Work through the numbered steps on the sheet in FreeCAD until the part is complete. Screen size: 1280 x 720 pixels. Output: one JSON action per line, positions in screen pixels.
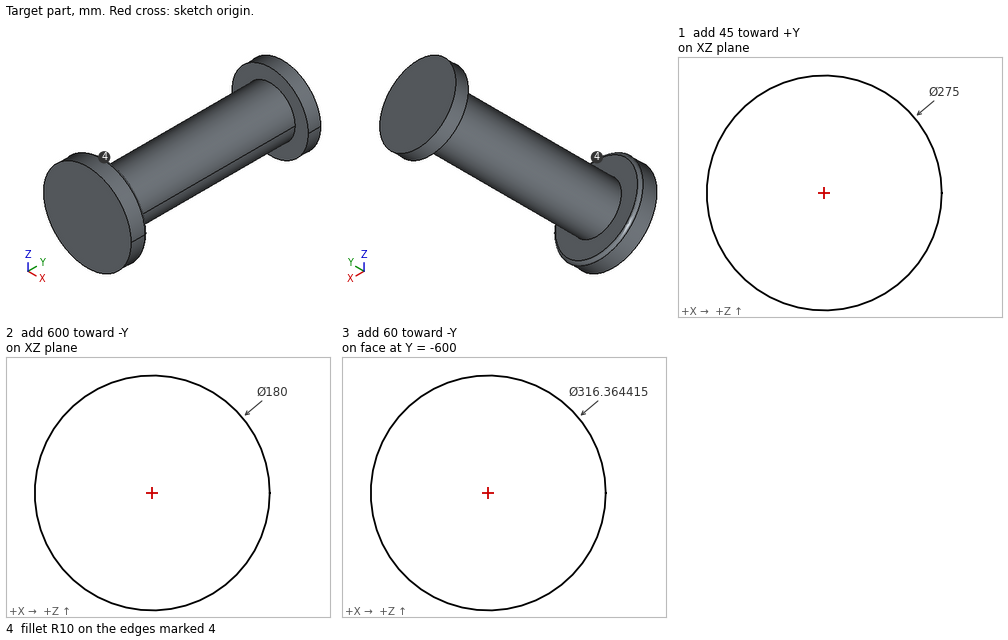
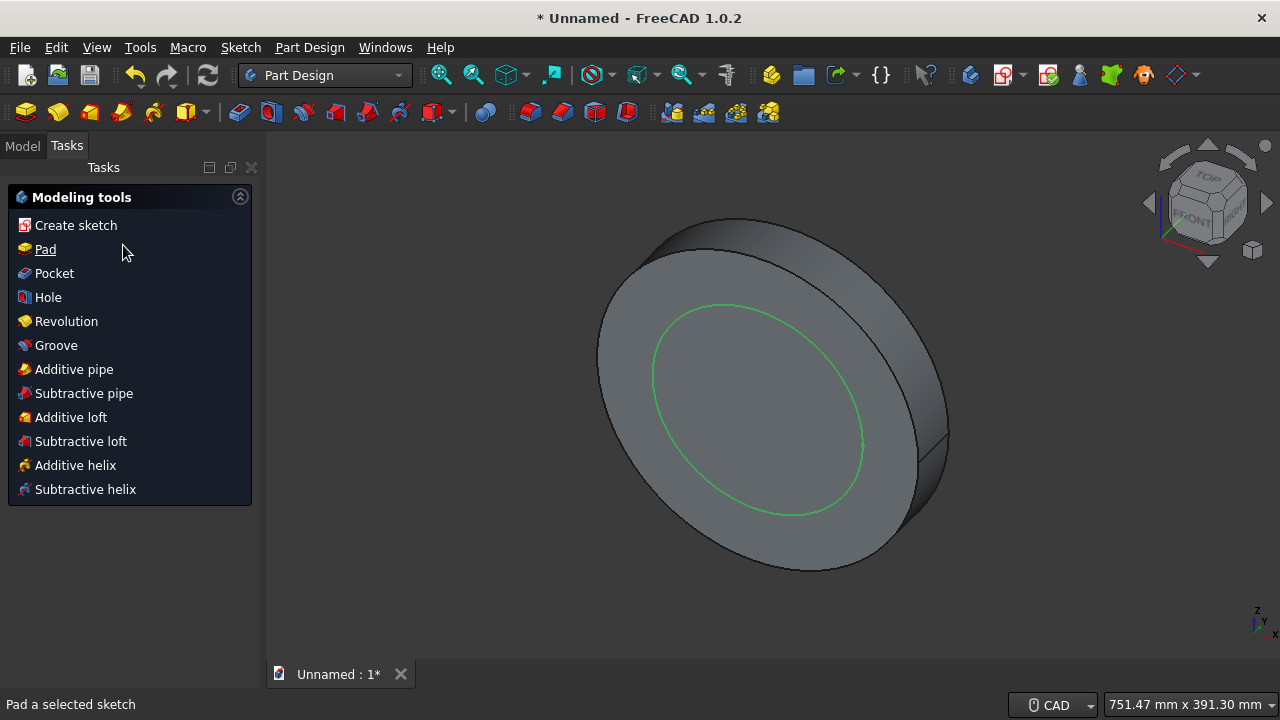
{"action": "left_click", "coordinate": [26, 112]}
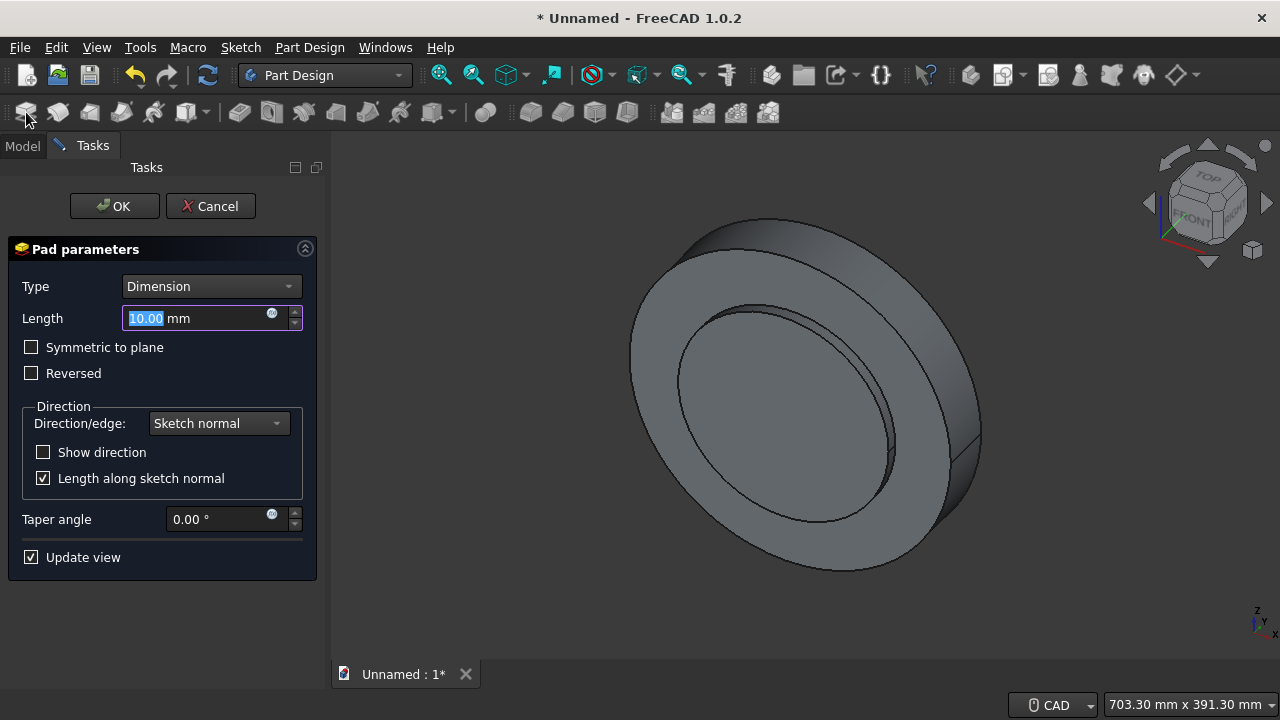
{"action": "type", "text": "600"}
{"action": "key", "text": "Tab"}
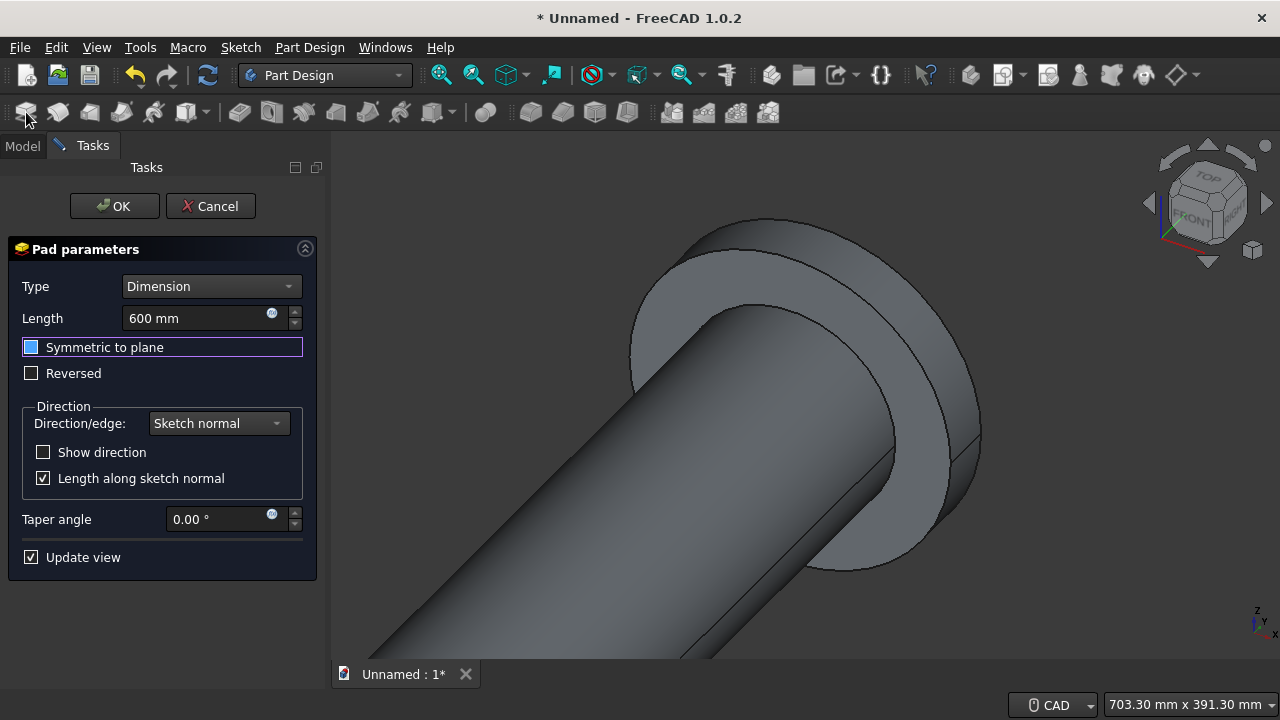
{"action": "left_click", "coordinate": [115, 206]}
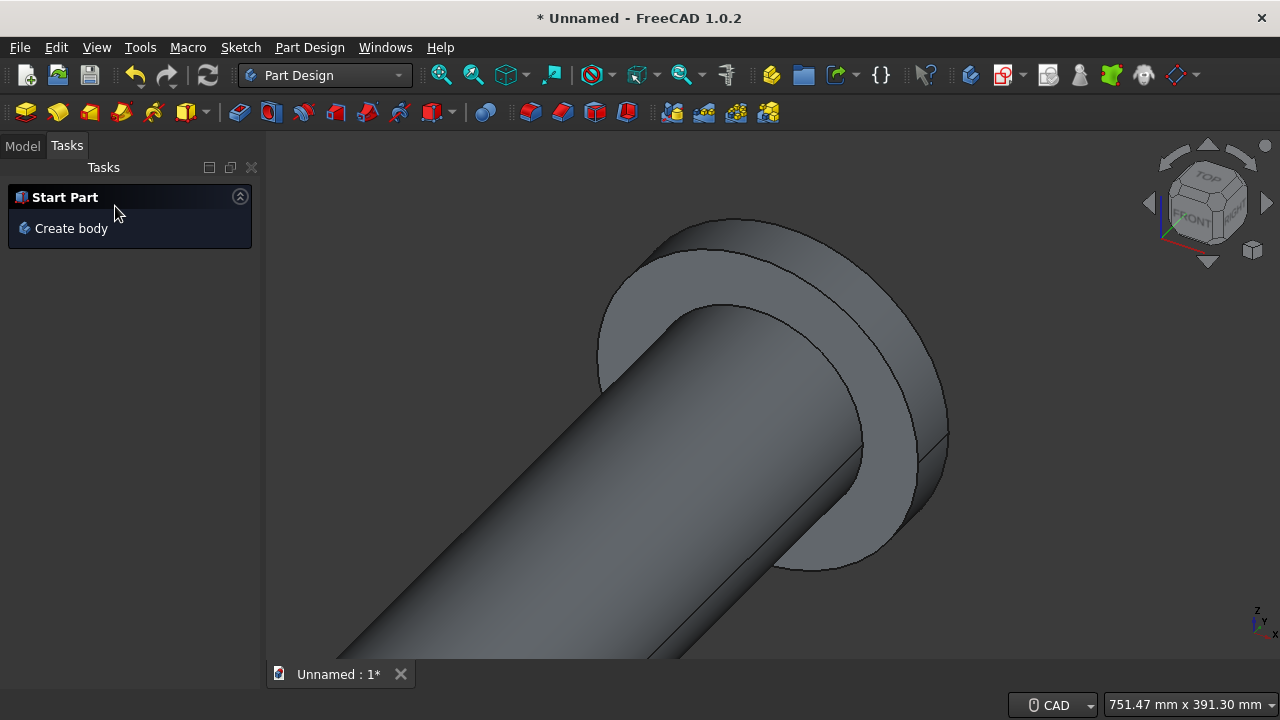
{"action": "left_click", "coordinate": [442, 76]}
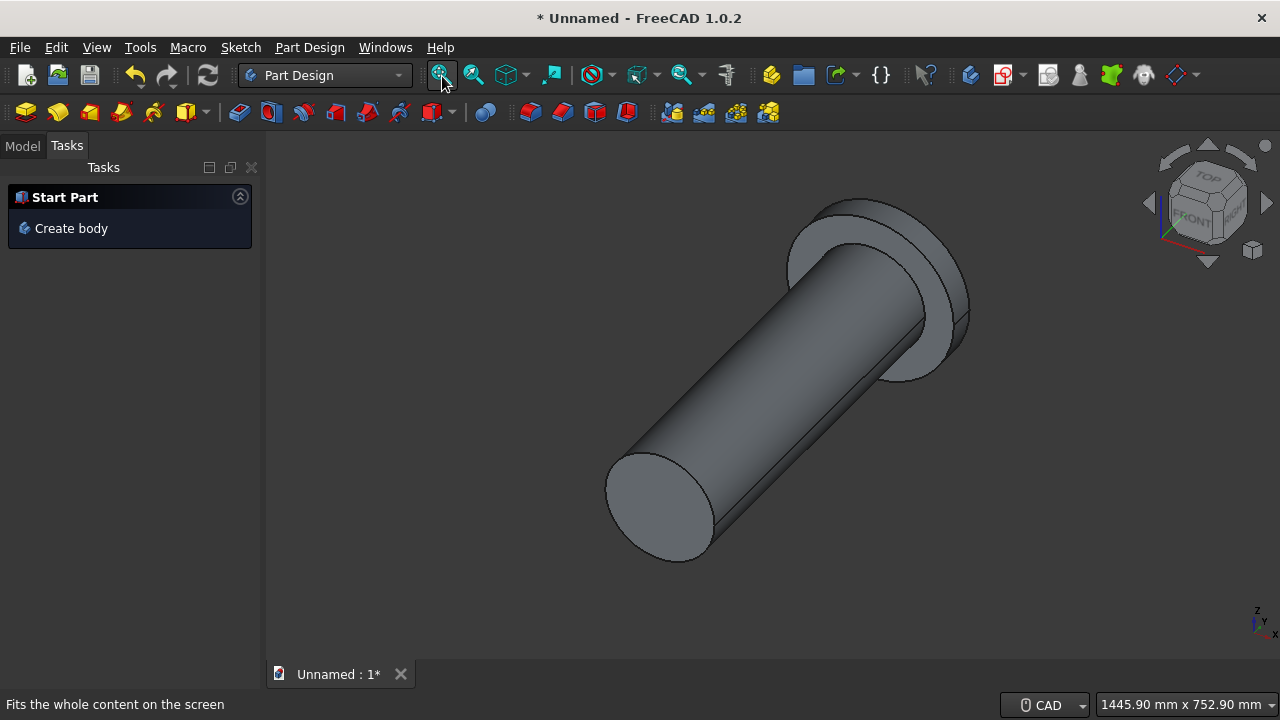
{"action": "left_click", "coordinate": [660, 506]}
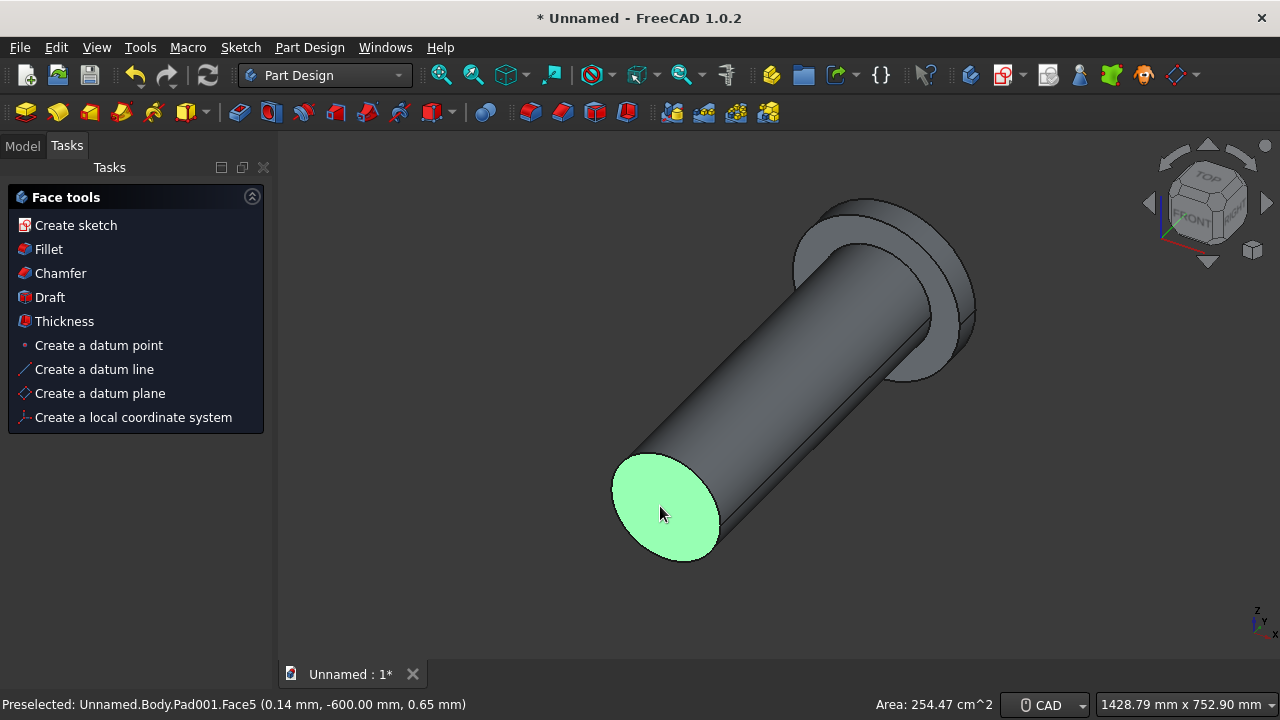
{"action": "left_click", "coordinate": [1004, 76]}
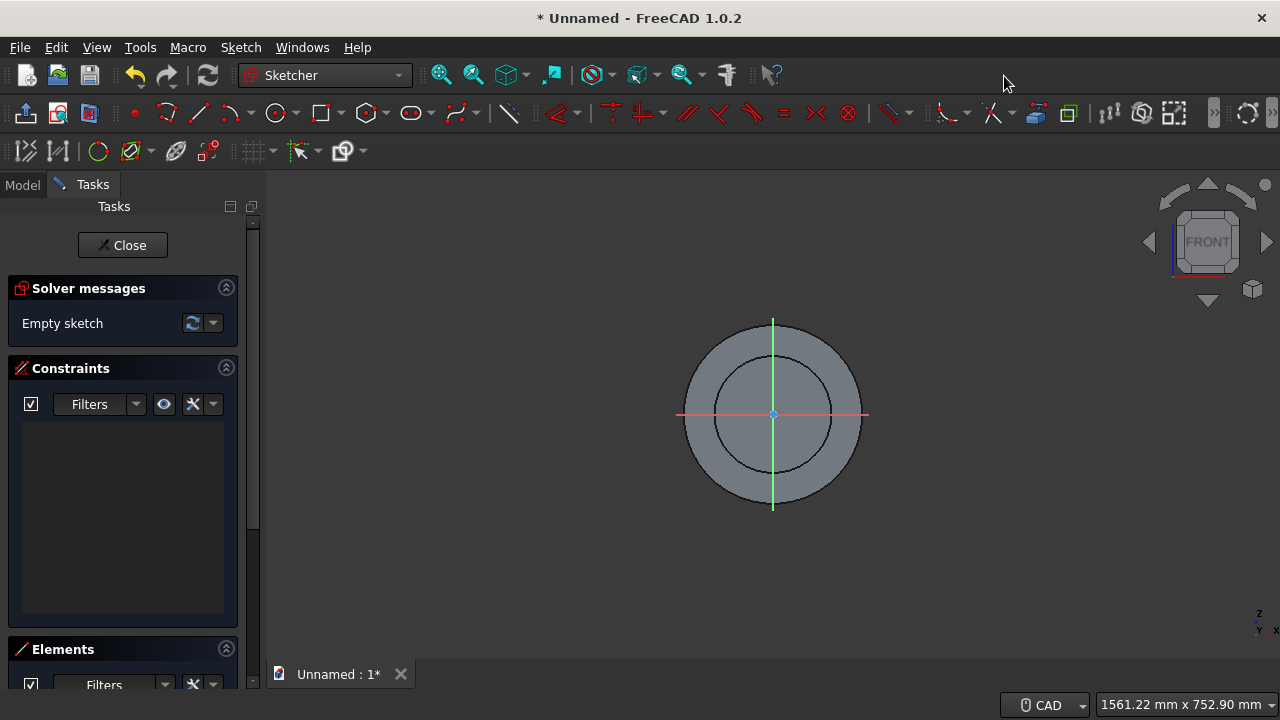
{"action": "scroll", "coordinate": [912, 414], "scroll_direction": "up", "scroll_amount": 2}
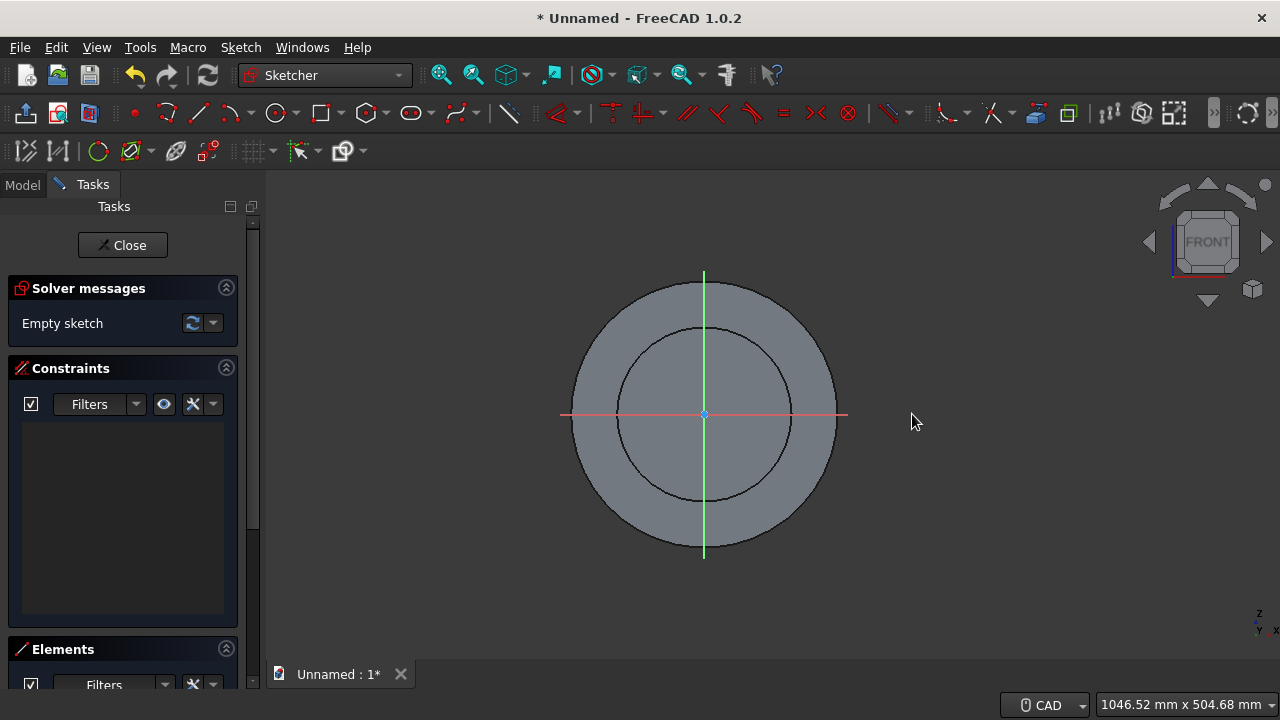
{"action": "key", "text": "g c"}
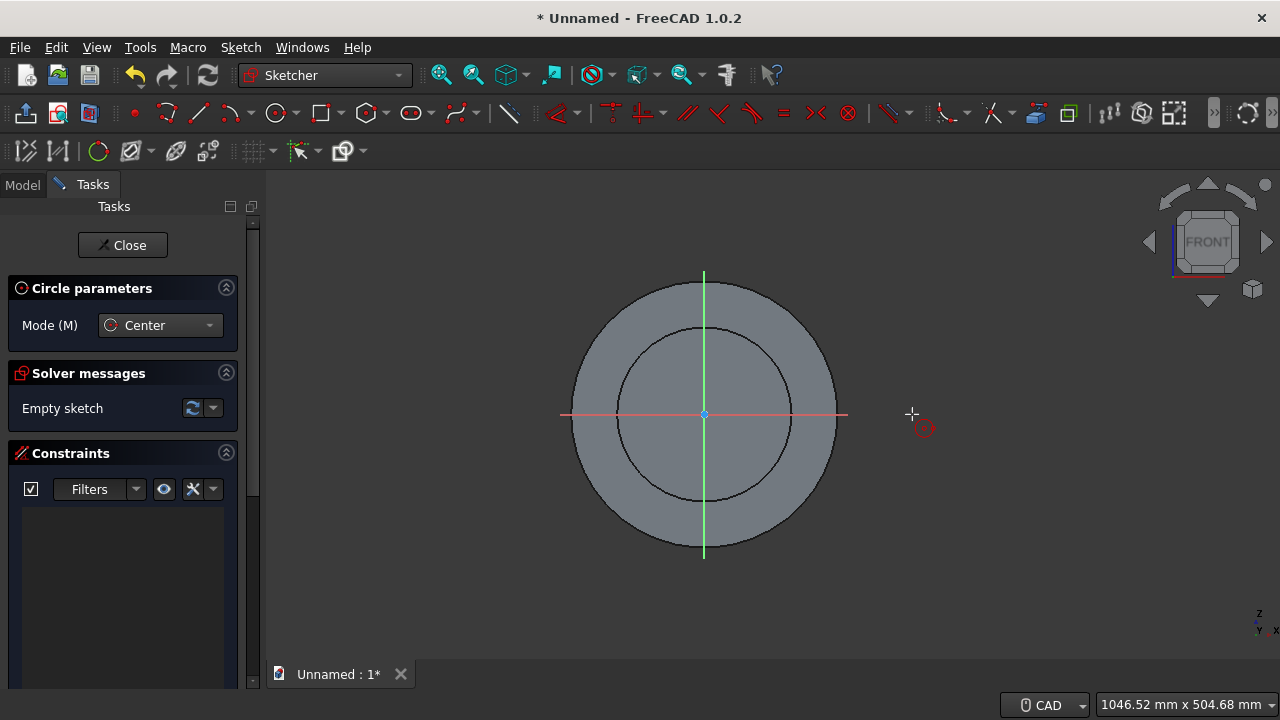
{"action": "left_click", "coordinate": [704, 414]}
{"action": "mouse_move", "coordinate": [813, 306]}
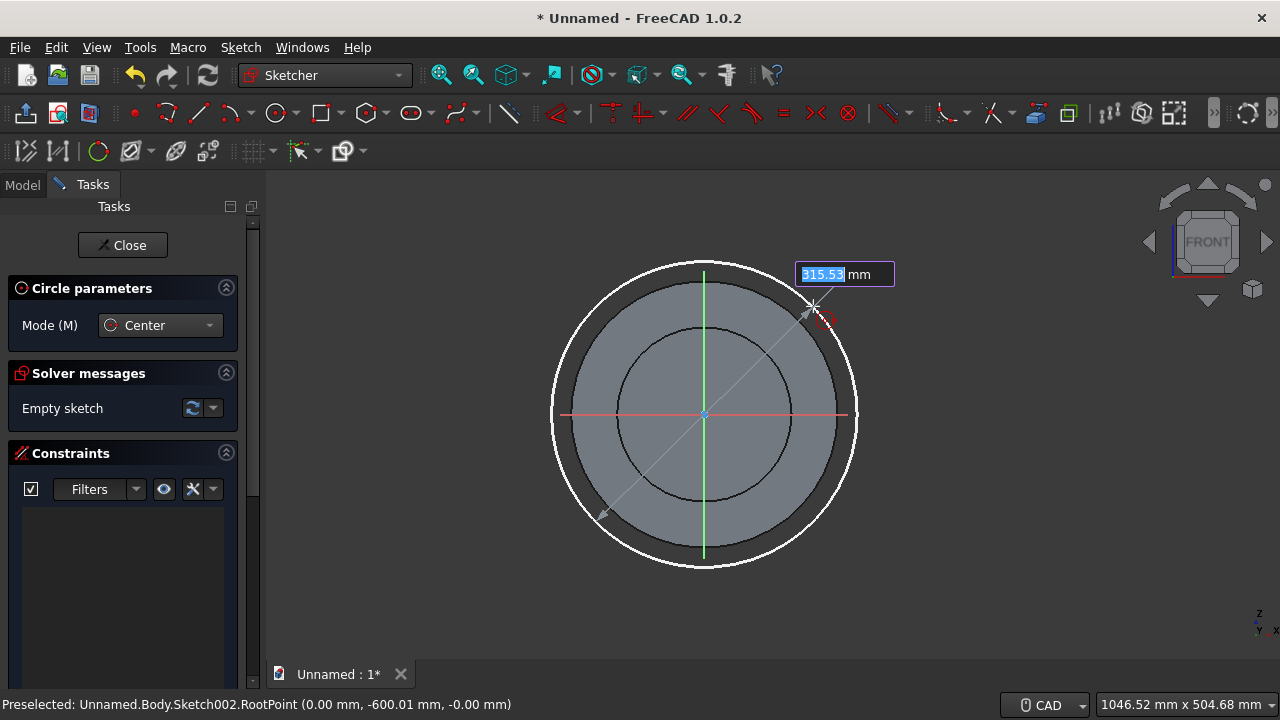
{"action": "type", "text": "316.364415"}
{"action": "key", "text": "Return"}
{"action": "key", "text": "Escape"}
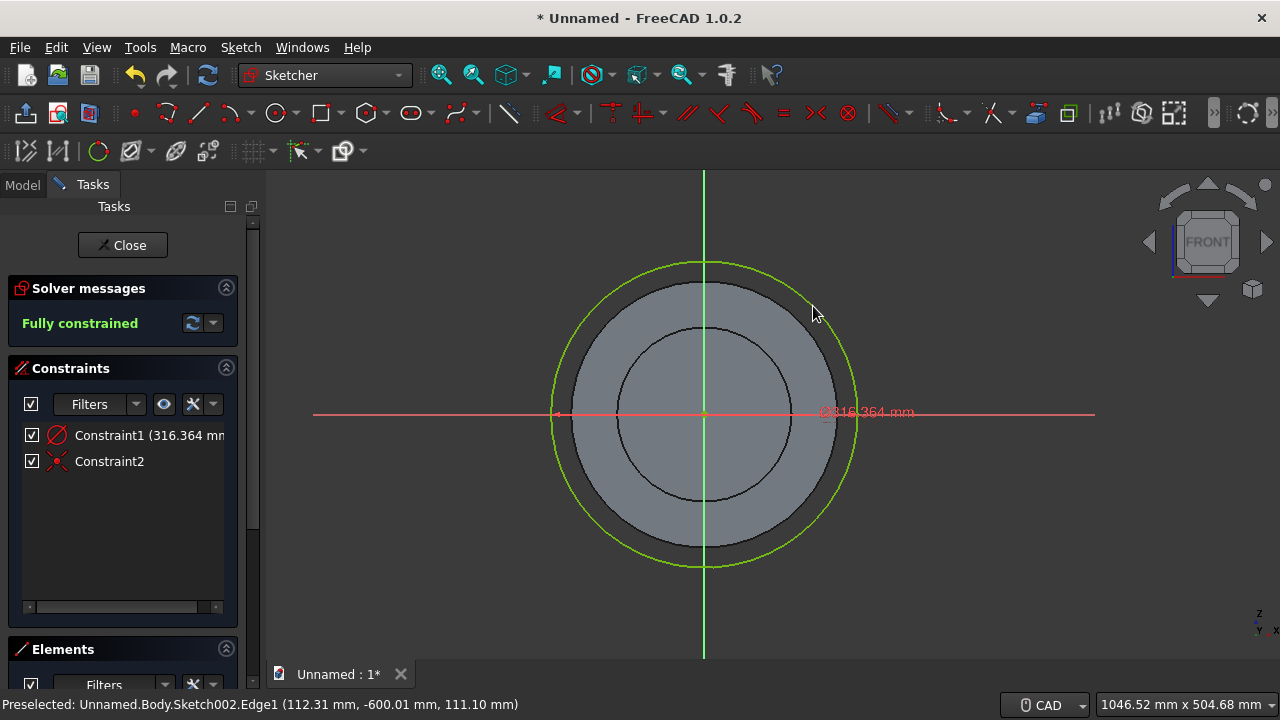
{"action": "left_click", "coordinate": [123, 245]}